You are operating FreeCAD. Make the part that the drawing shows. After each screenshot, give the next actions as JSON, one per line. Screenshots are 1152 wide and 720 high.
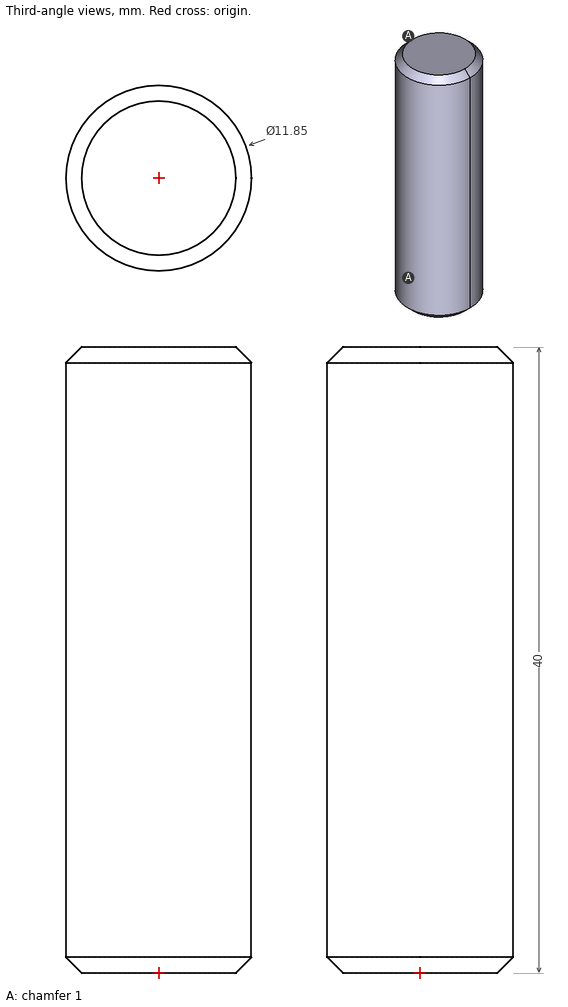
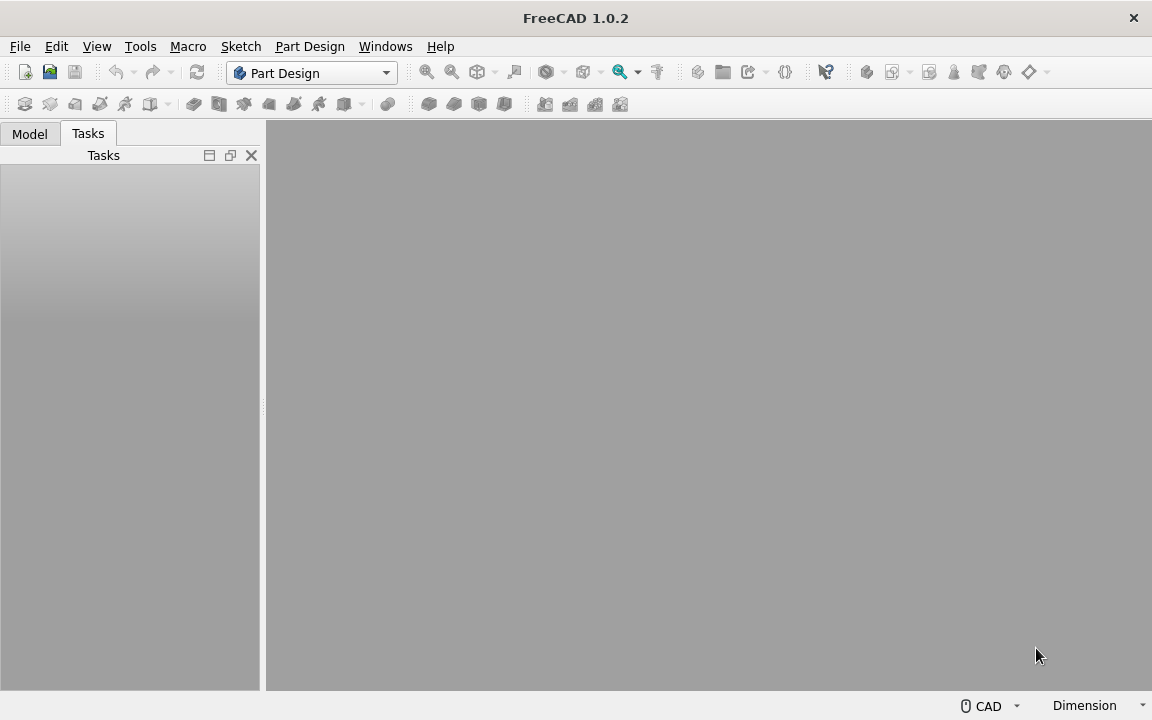
{"action": "left_click", "coordinate": [25, 72]}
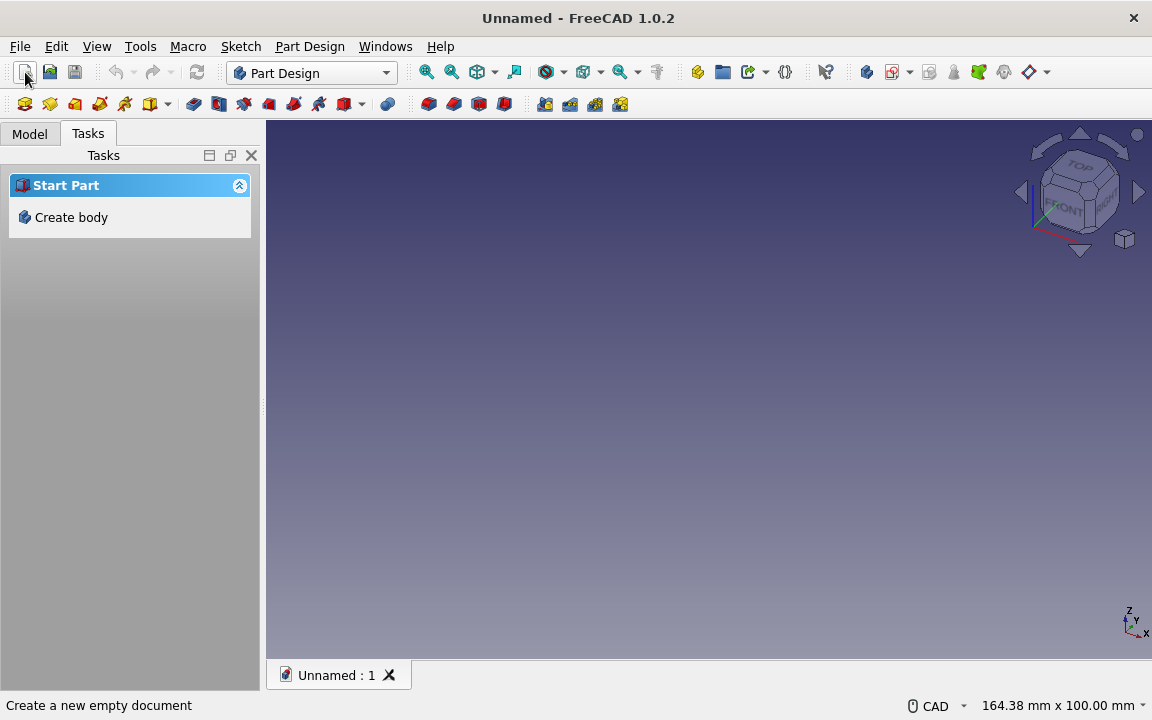
{"action": "left_click", "coordinate": [892, 72]}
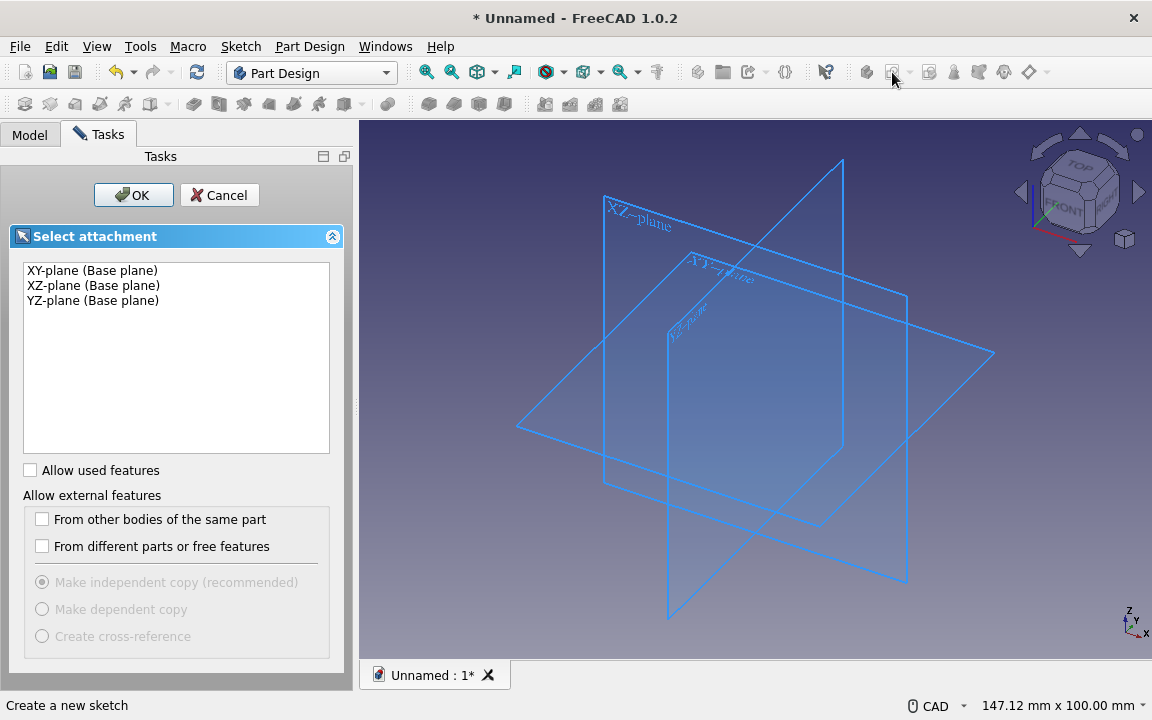
{"action": "left_click", "coordinate": [84, 270]}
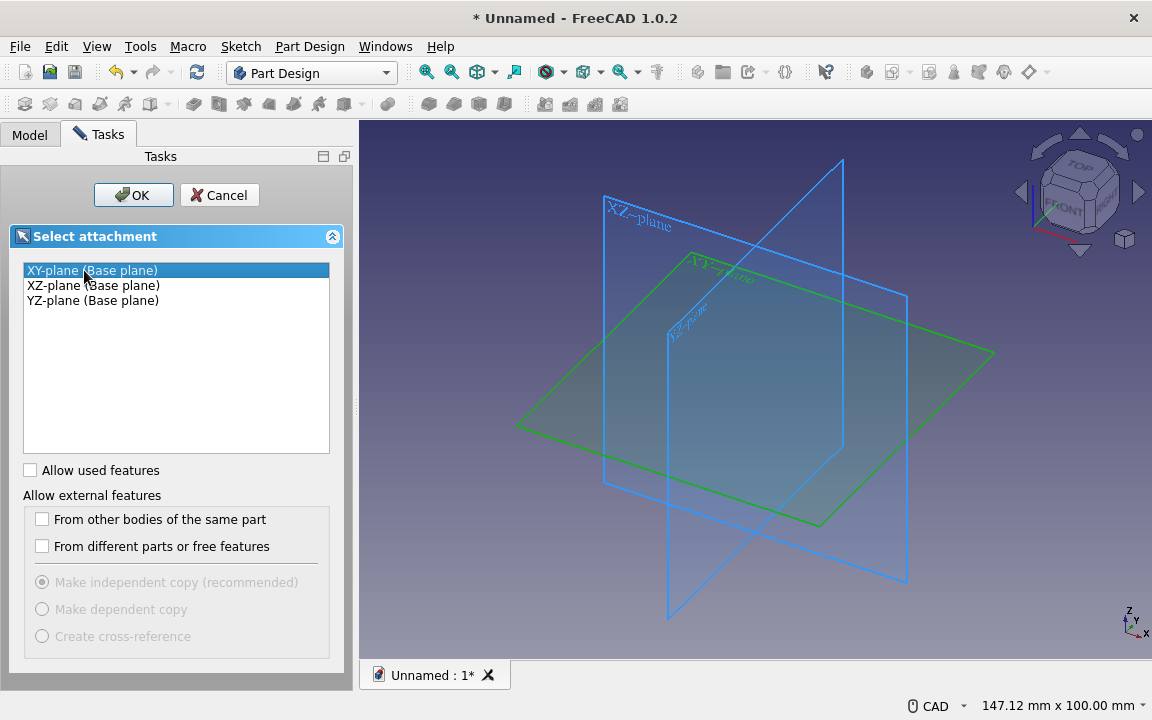
{"action": "left_click", "coordinate": [134, 195]}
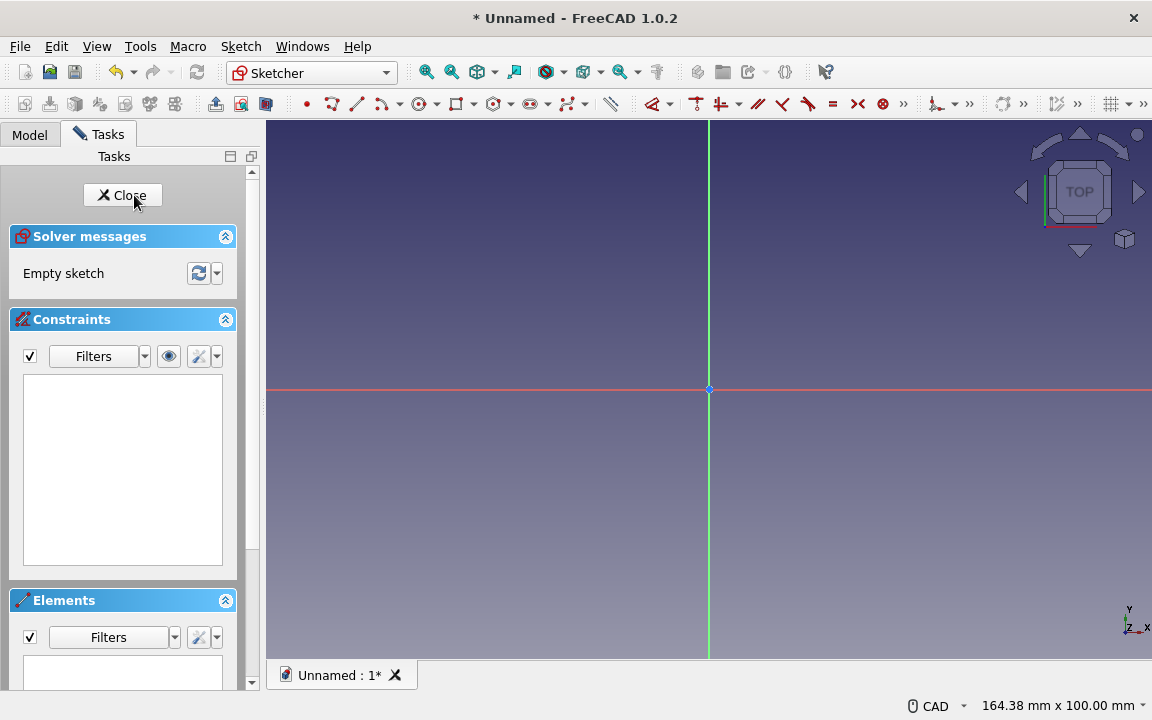
{"action": "scroll", "coordinate": [726, 390], "scroll_direction": "up", "scroll_amount": 8}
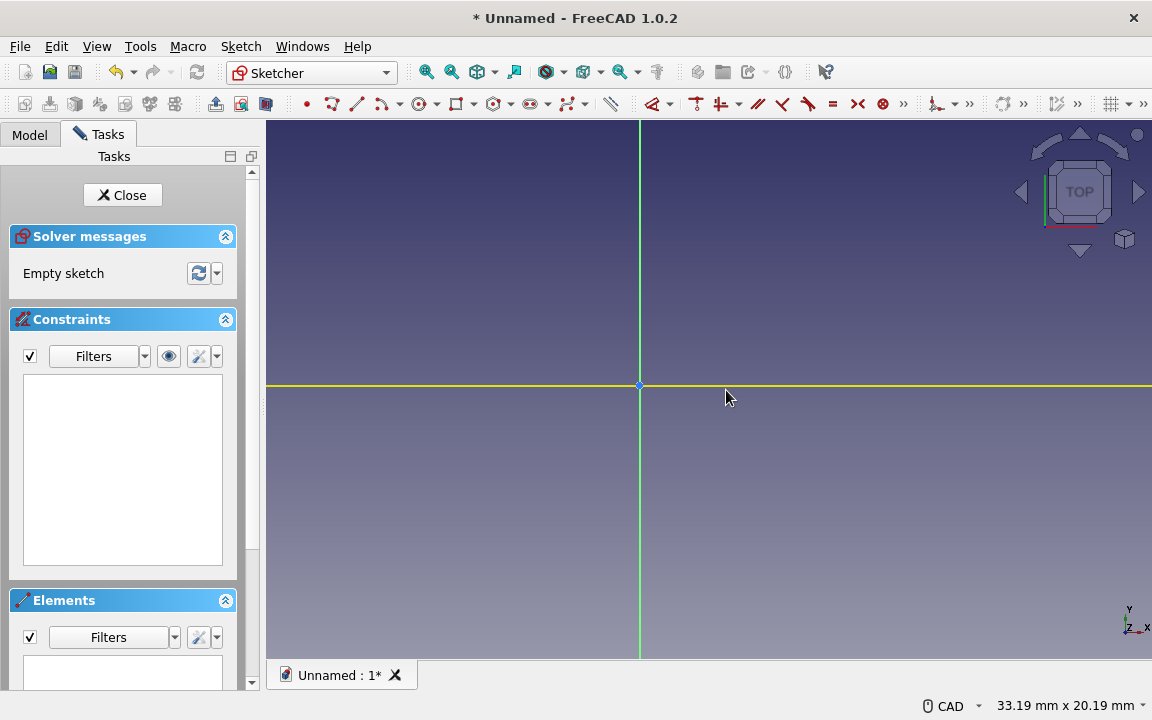
{"action": "left_click", "coordinate": [418, 104]}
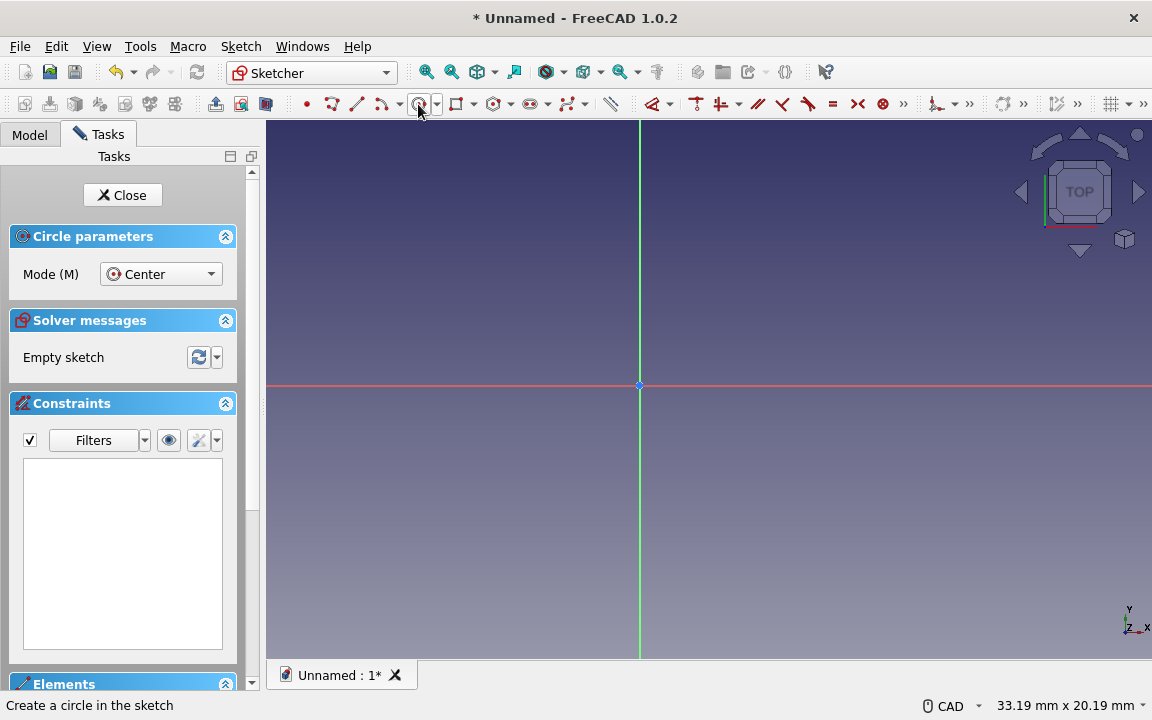
{"action": "left_click", "coordinate": [640, 386]}
{"action": "mouse_move", "coordinate": [752, 274]}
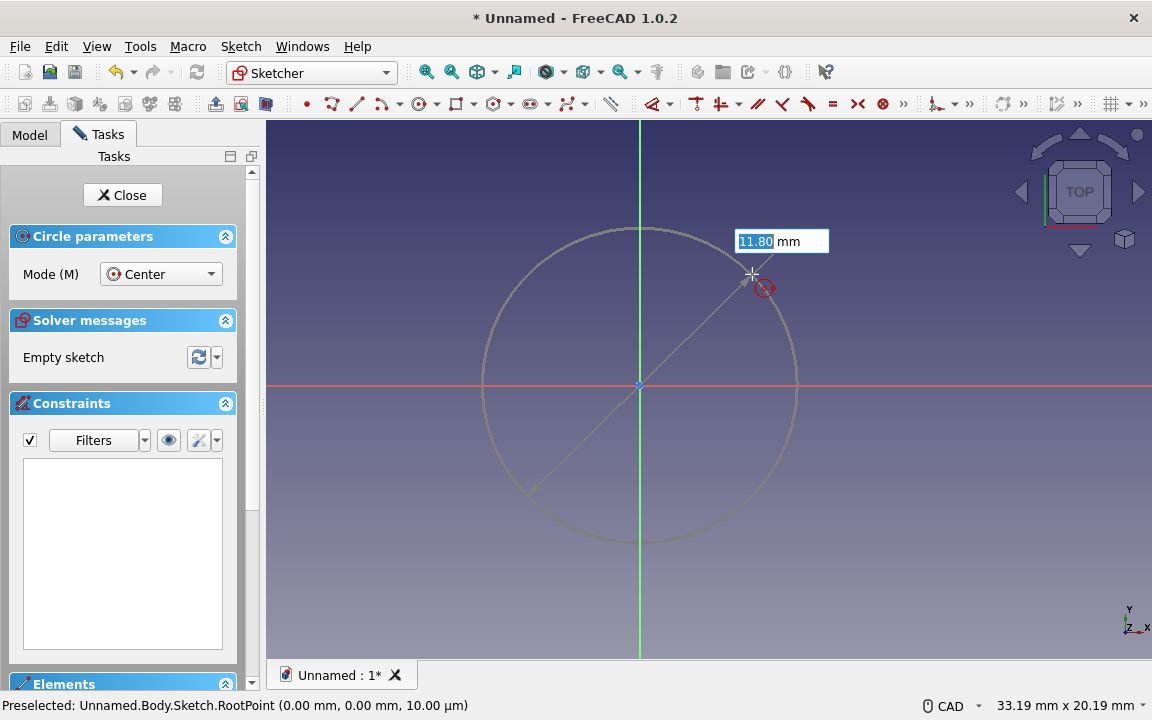
{"action": "type", "text": "11.85"}
{"action": "key", "text": "Return"}
{"action": "key", "text": "Escape"}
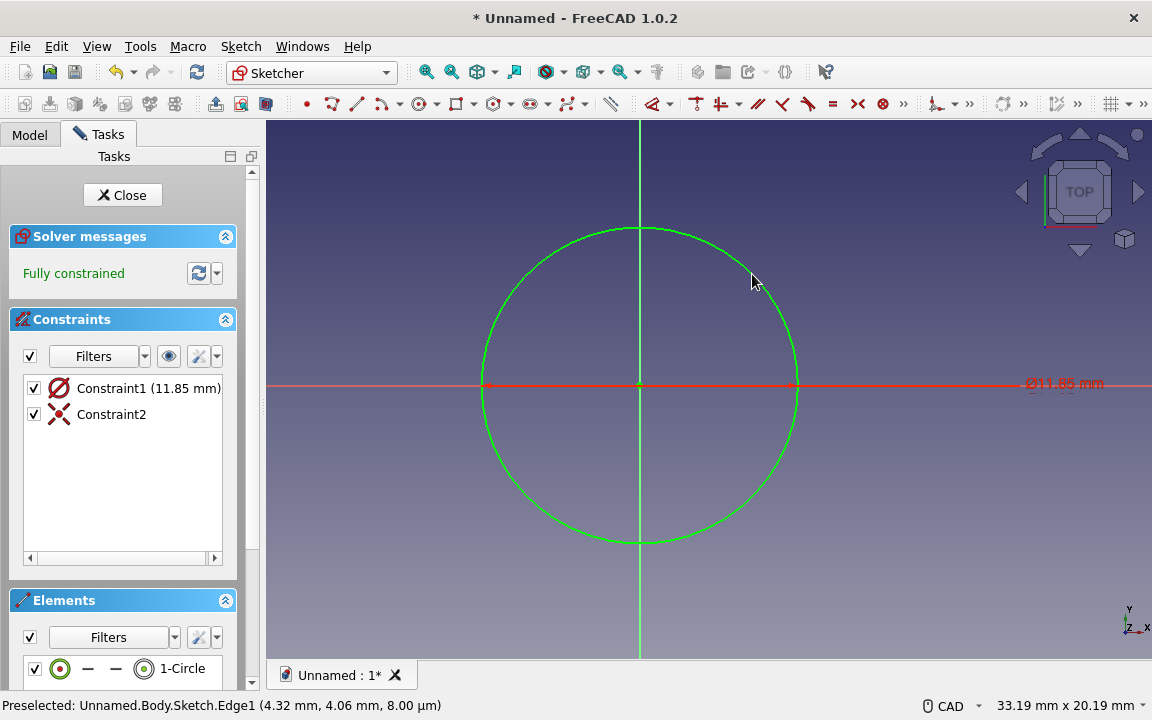
{"action": "left_click", "coordinate": [123, 195]}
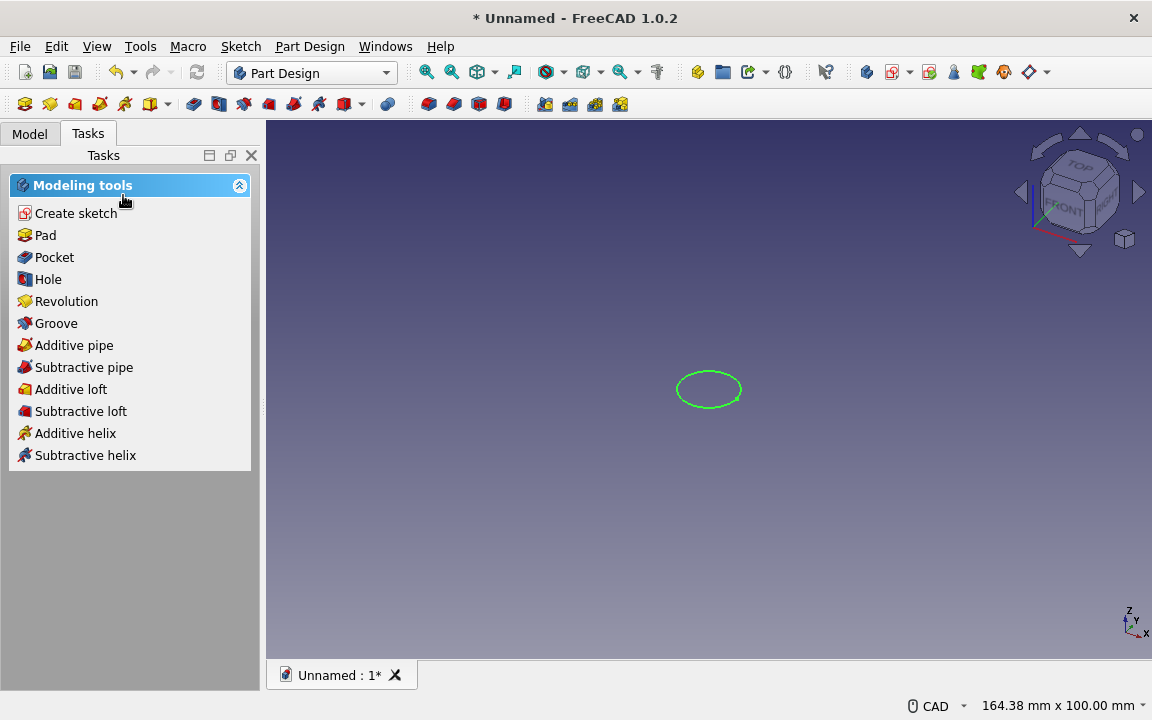
{"action": "left_click", "coordinate": [25, 104]}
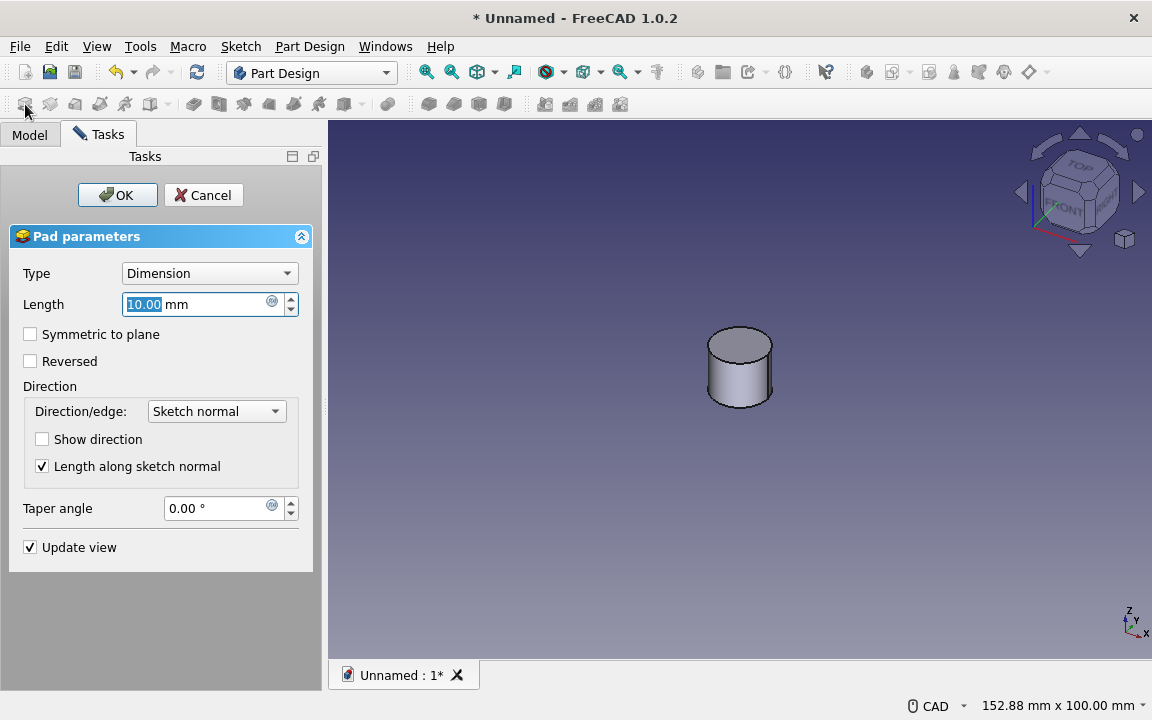
{"action": "type", "text": "40"}
{"action": "key", "text": "Tab"}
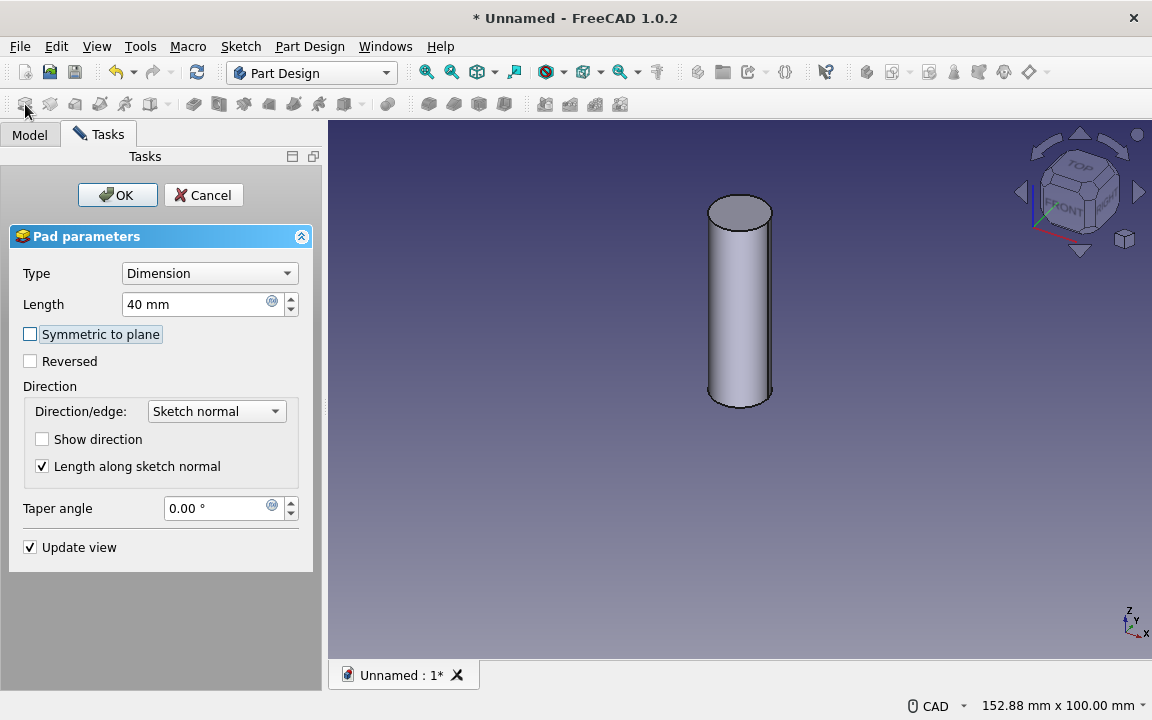
{"action": "left_click", "coordinate": [118, 195]}